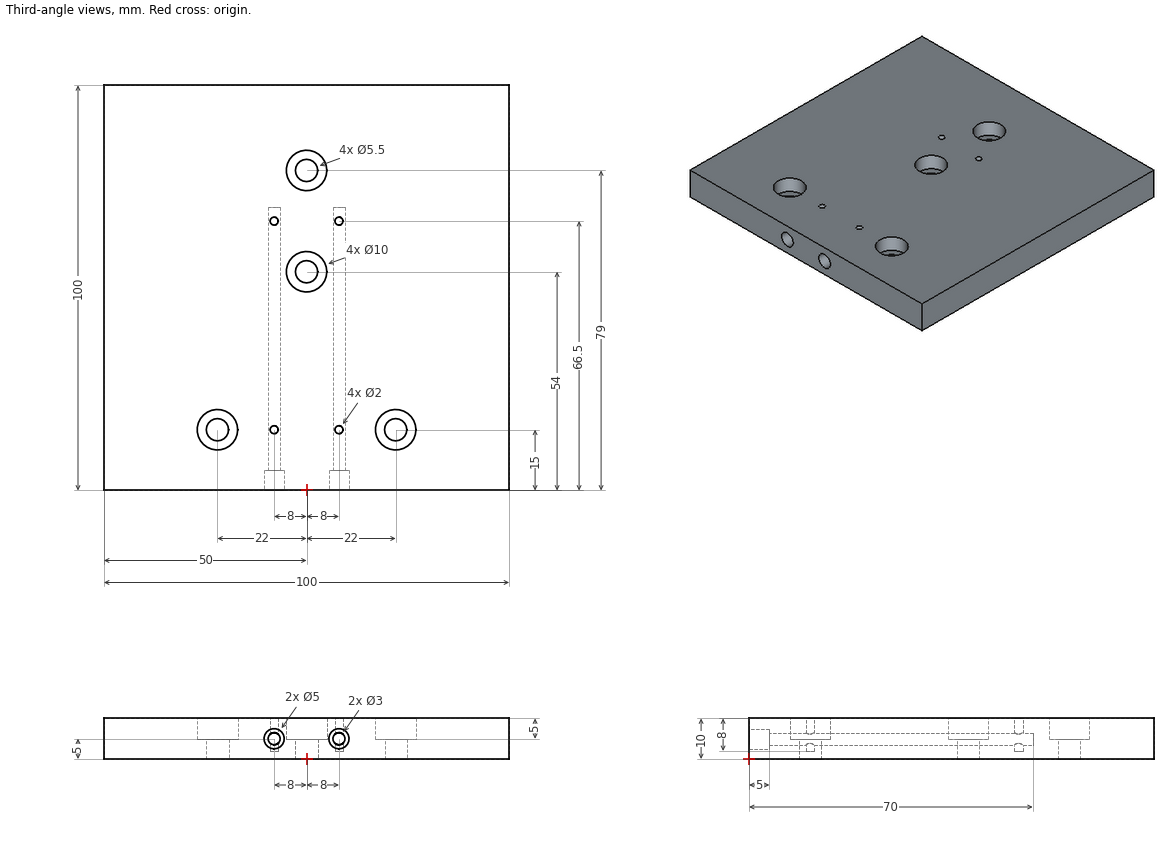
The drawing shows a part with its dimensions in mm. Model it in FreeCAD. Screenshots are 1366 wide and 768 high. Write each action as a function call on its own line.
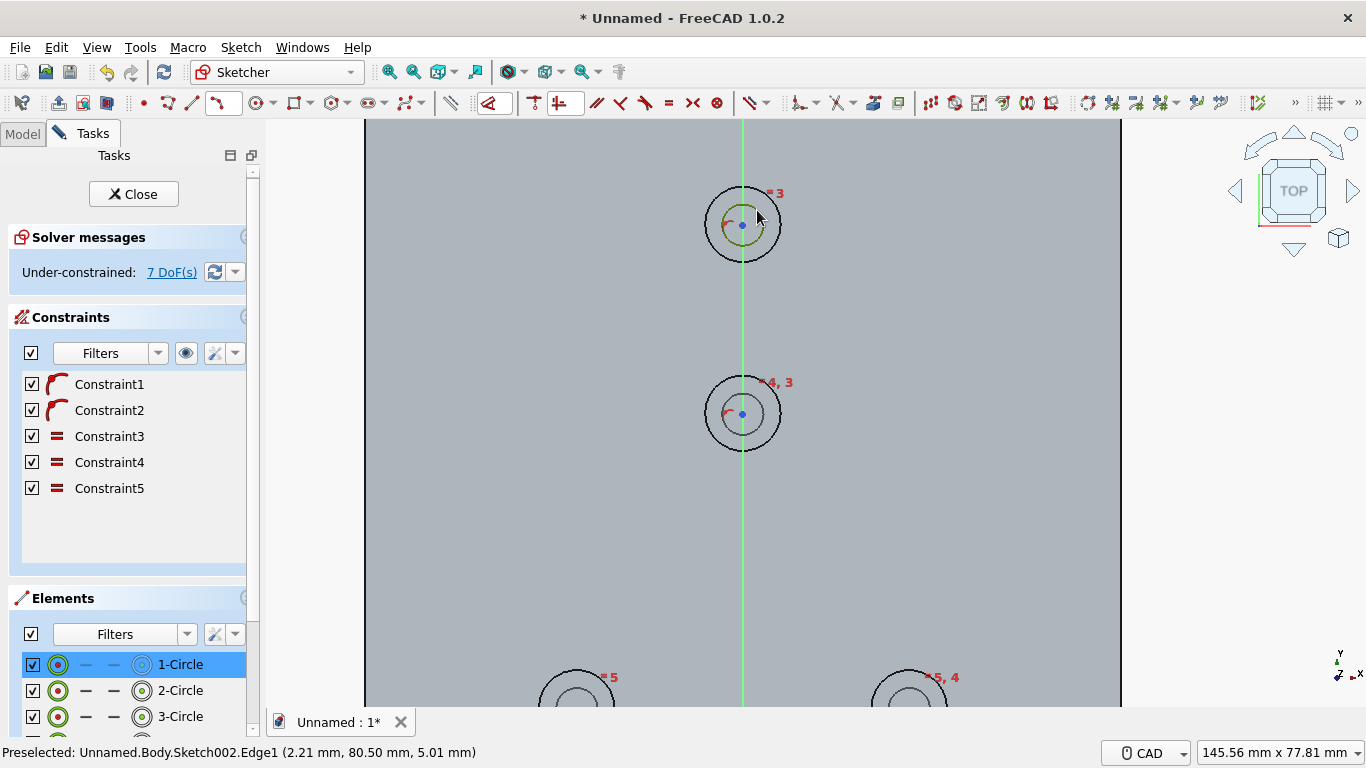
key(k)
key(o)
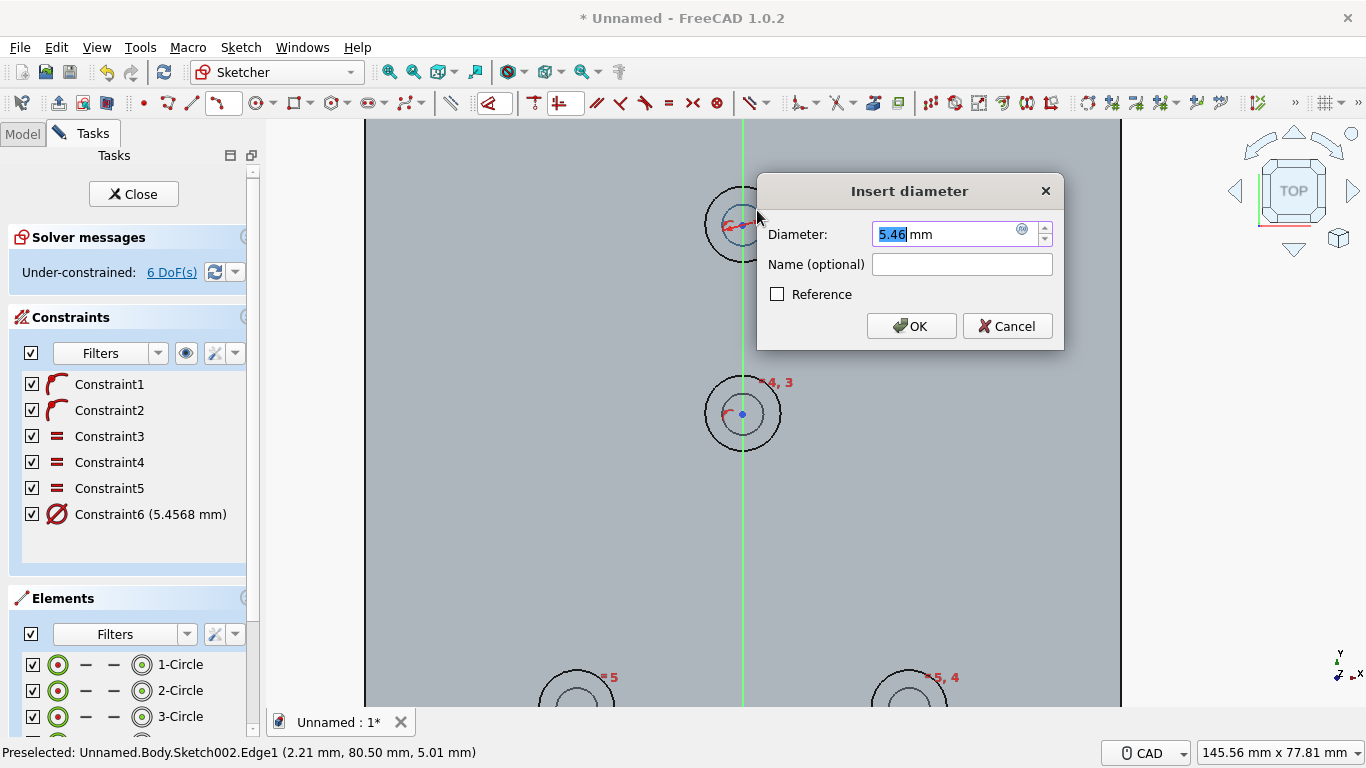
text(5.5)
key(Return)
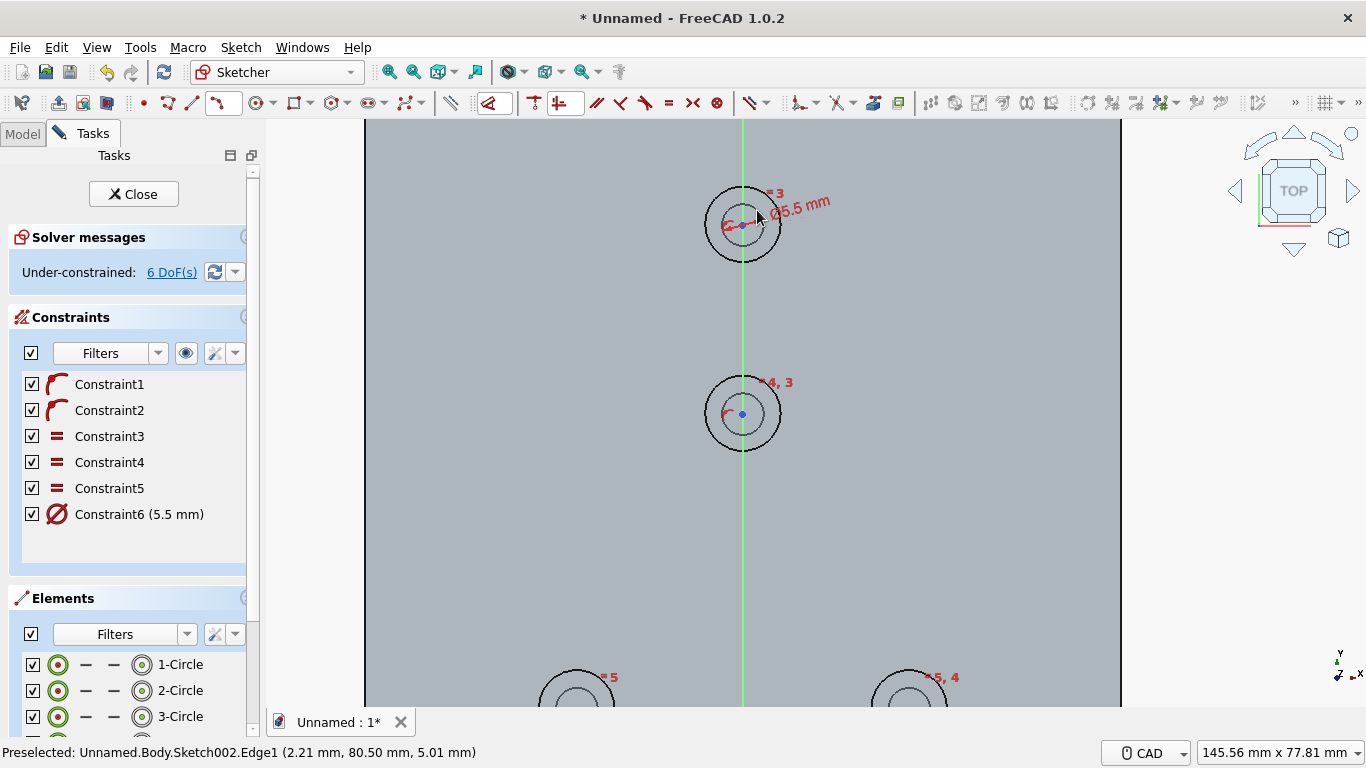
click(743, 225)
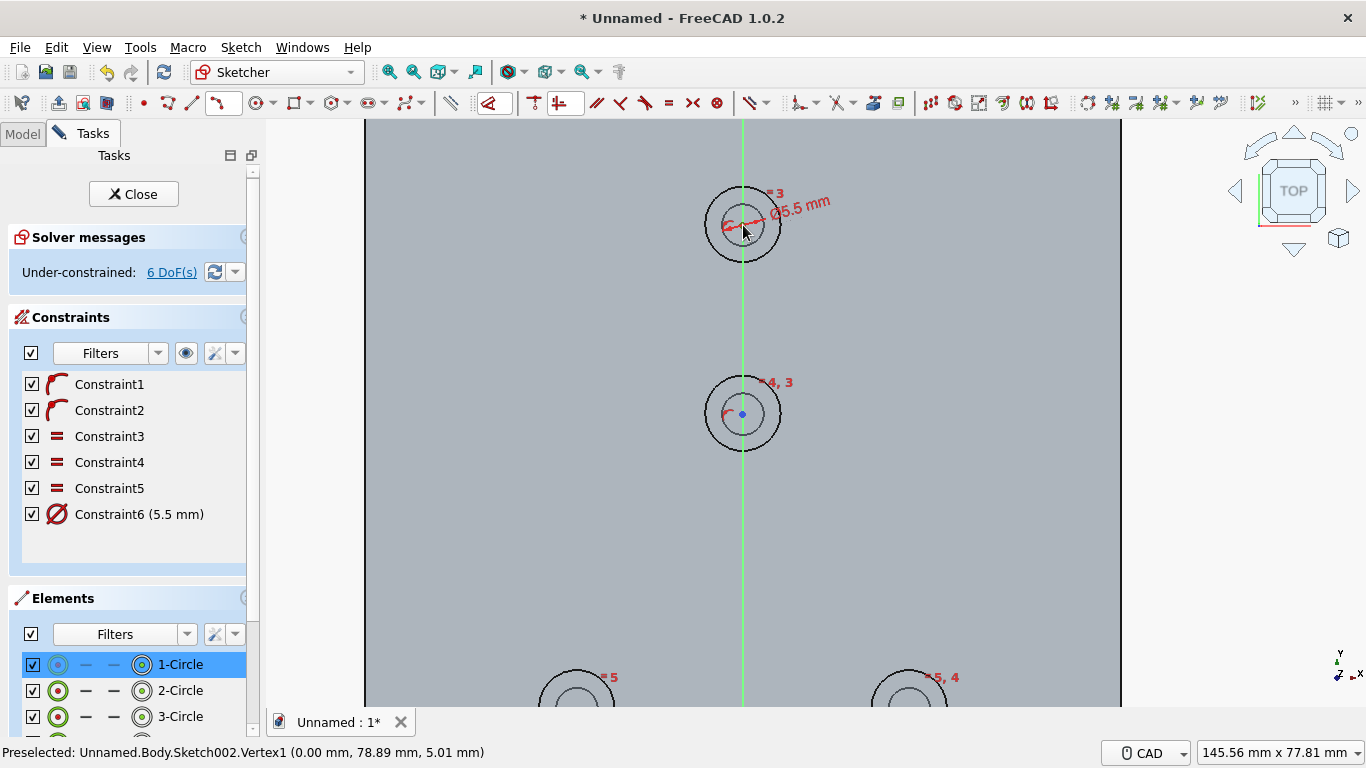
click(506, 104)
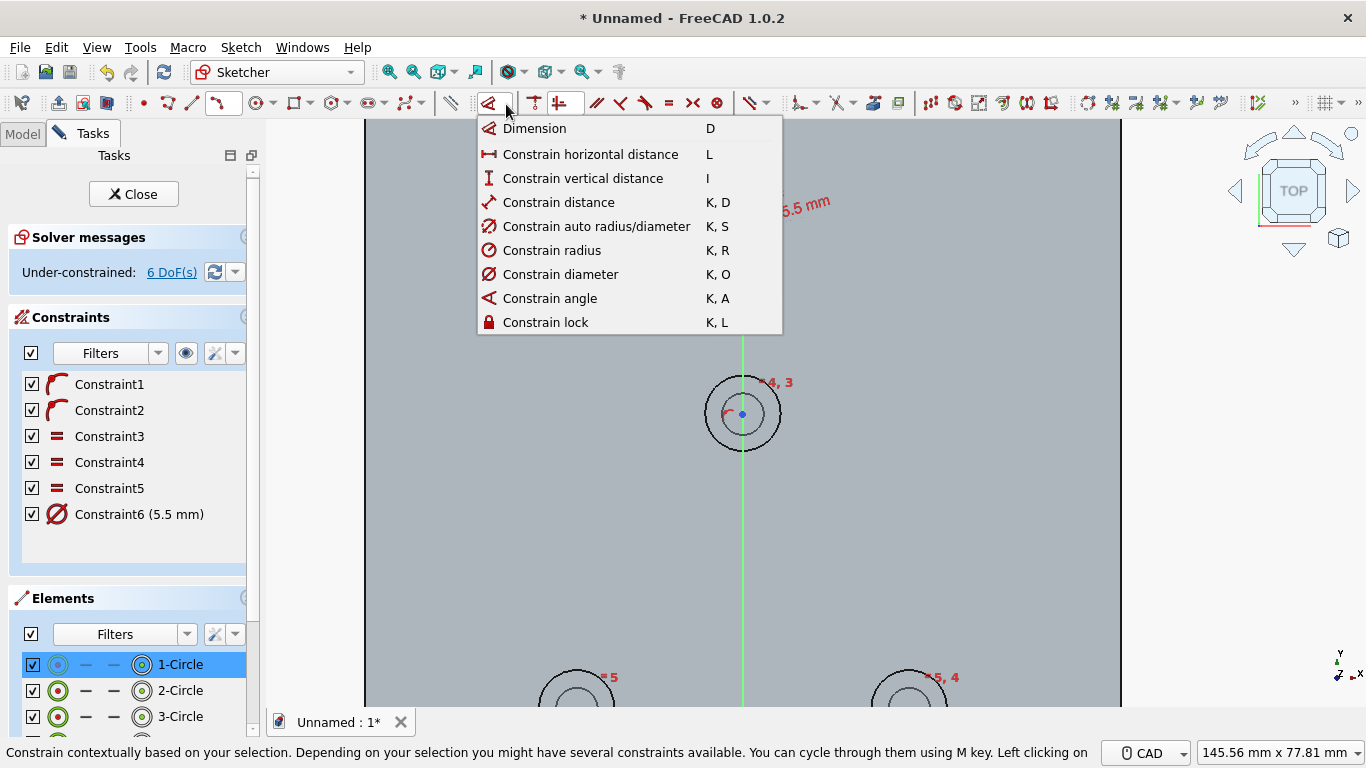
click(630, 178)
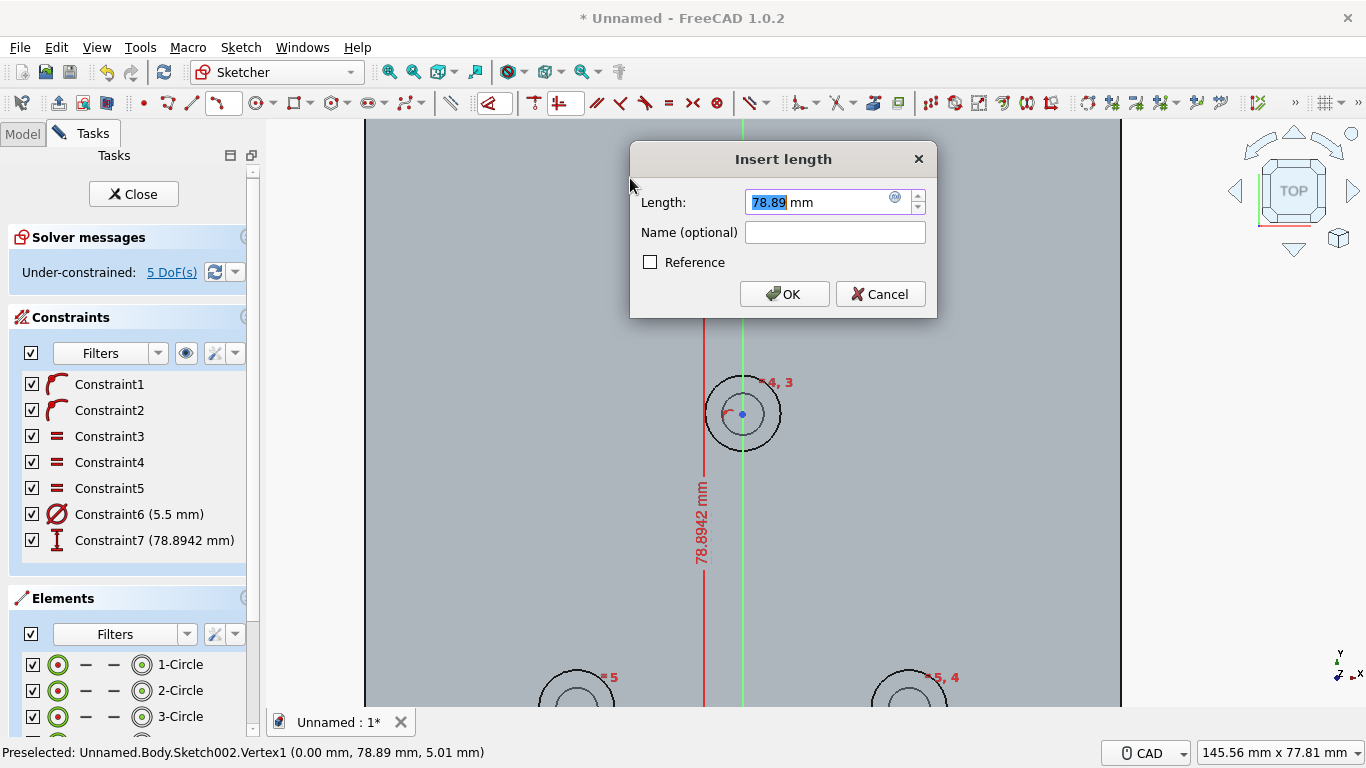
text(79)
key(Return)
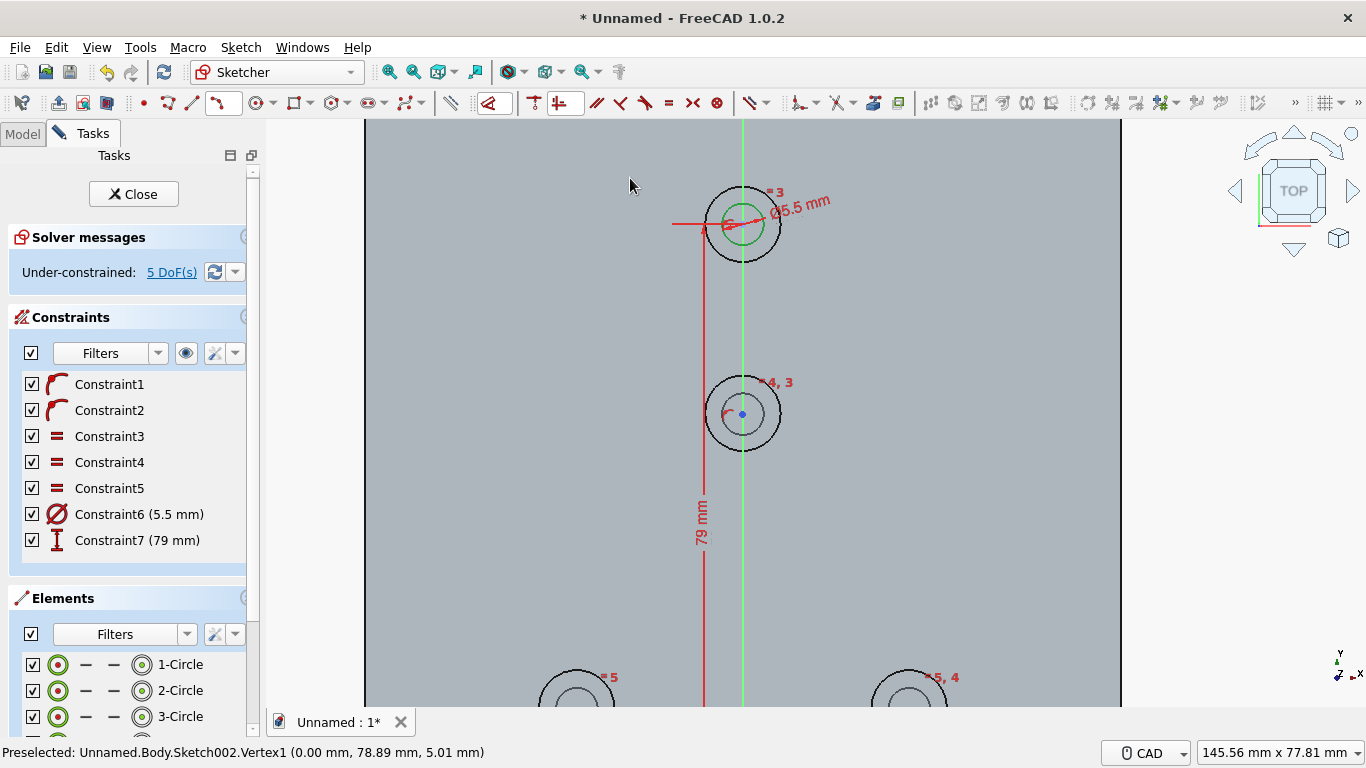
click(743, 414)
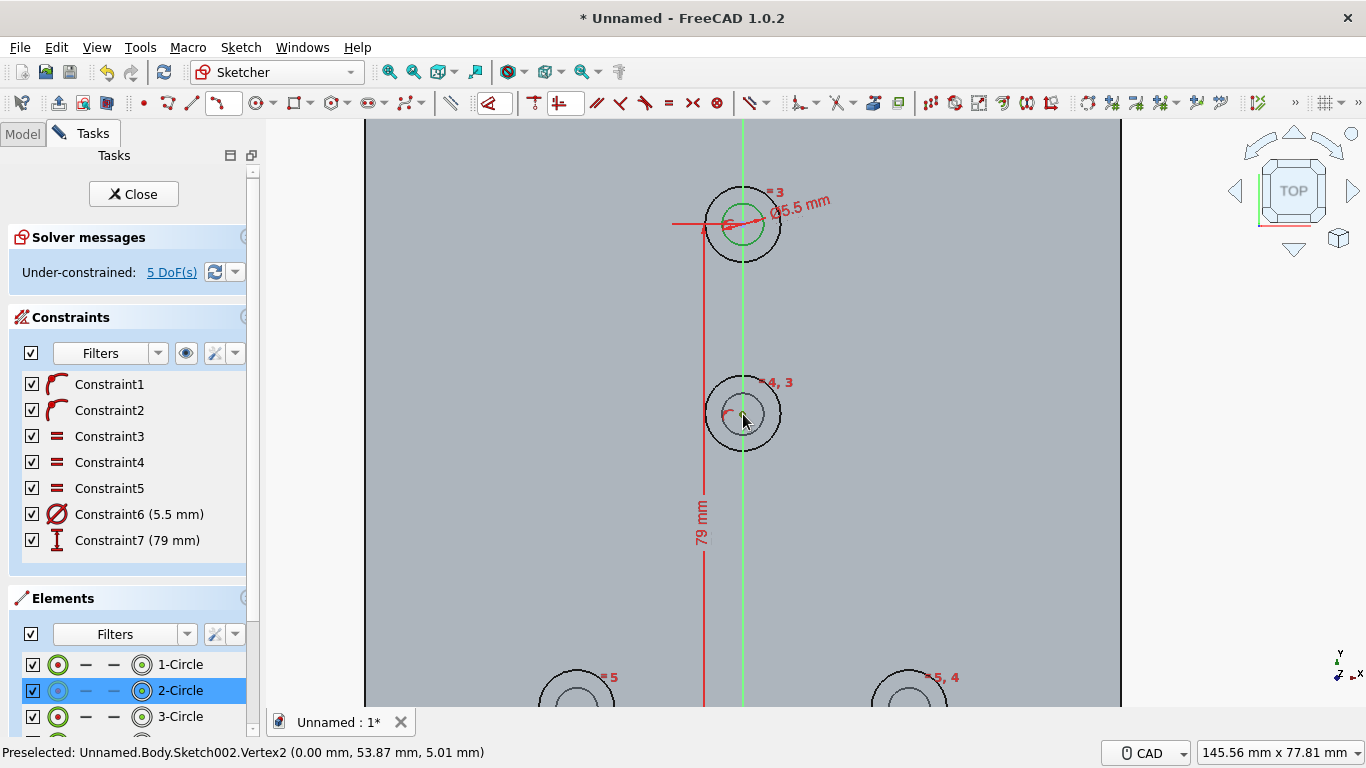
click(506, 104)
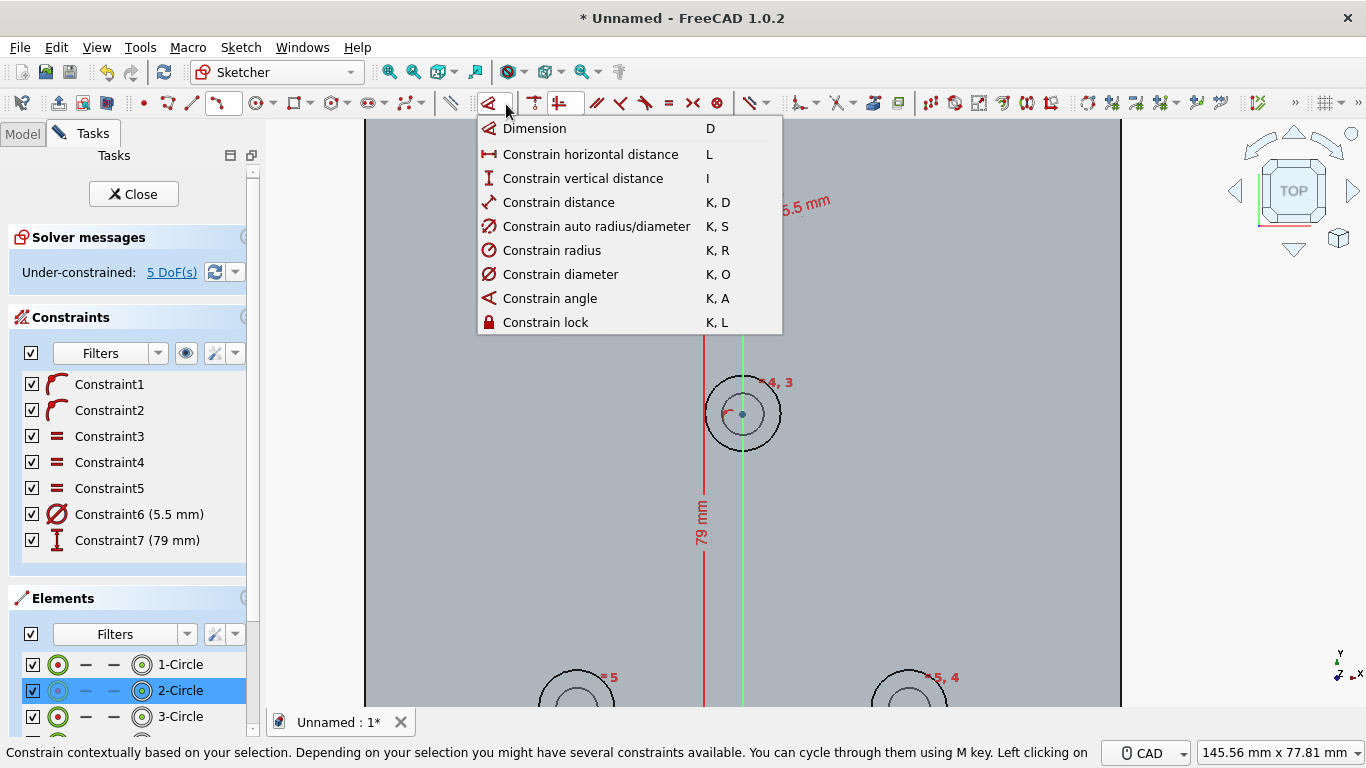
click(630, 178)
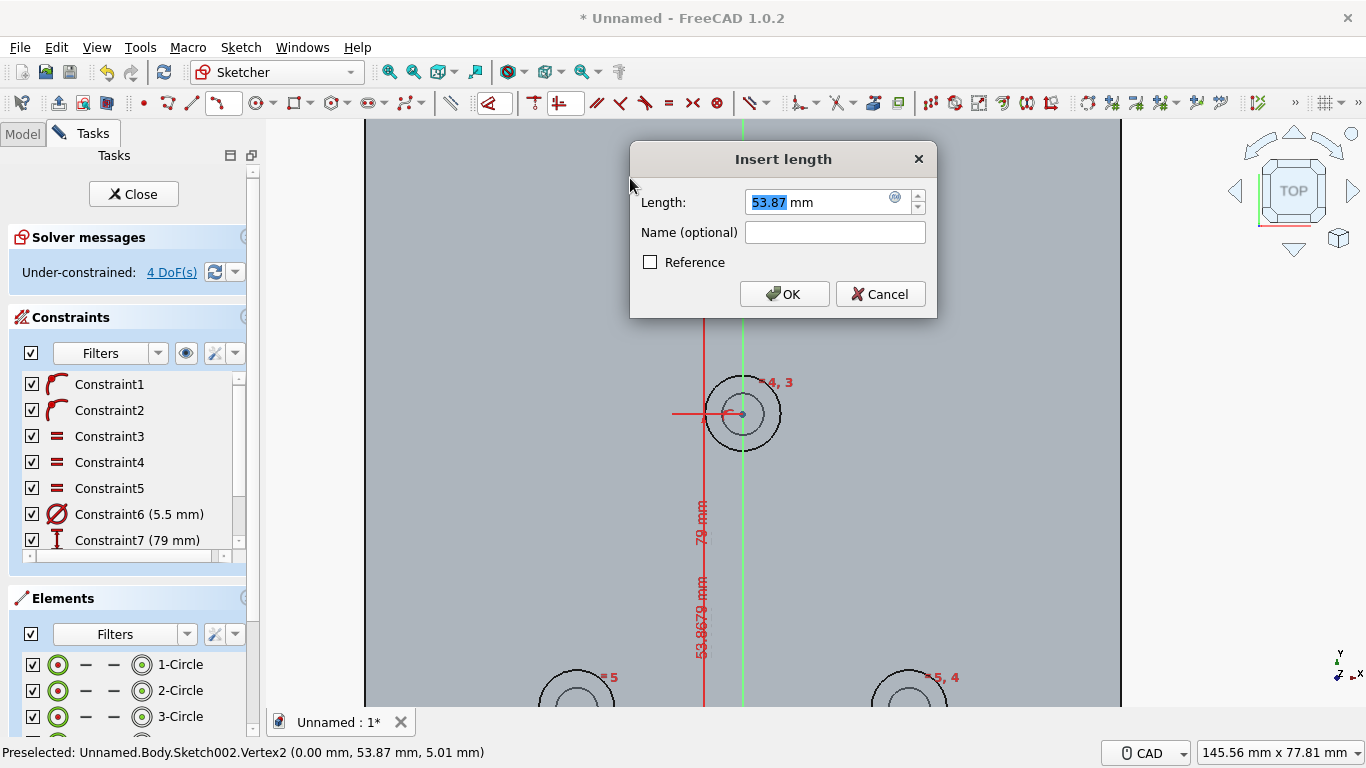
text(54)
key(Return)